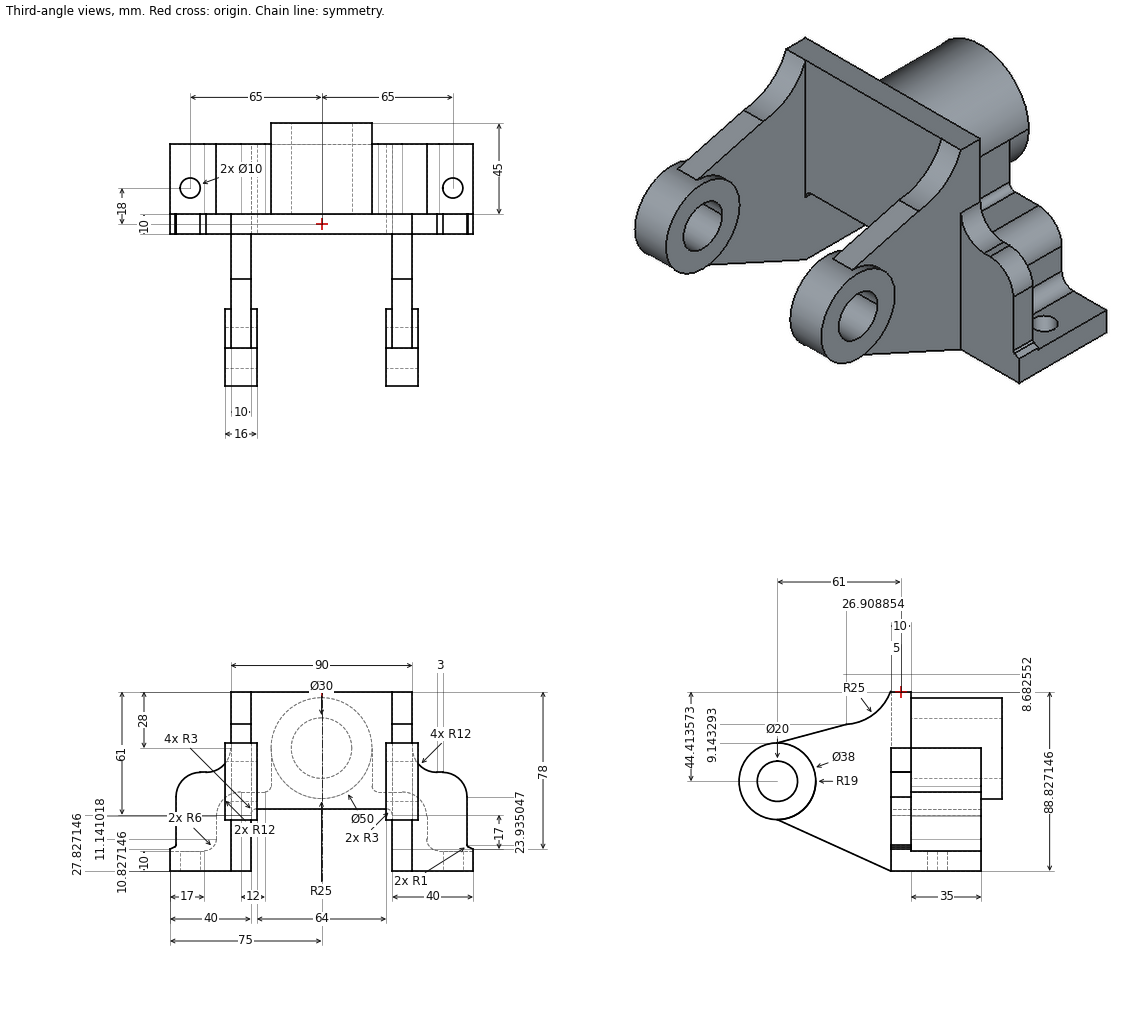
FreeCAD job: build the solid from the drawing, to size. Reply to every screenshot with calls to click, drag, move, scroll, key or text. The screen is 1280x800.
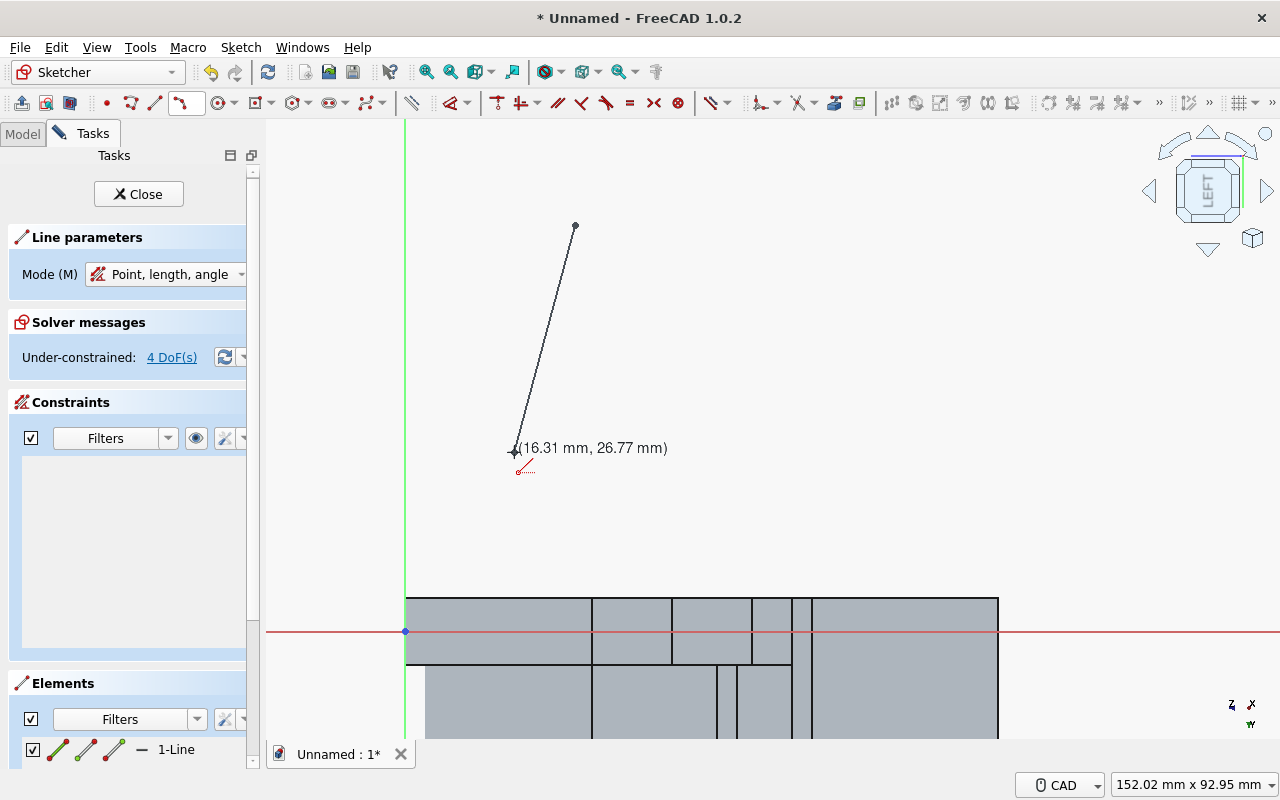
key(g)
key(m)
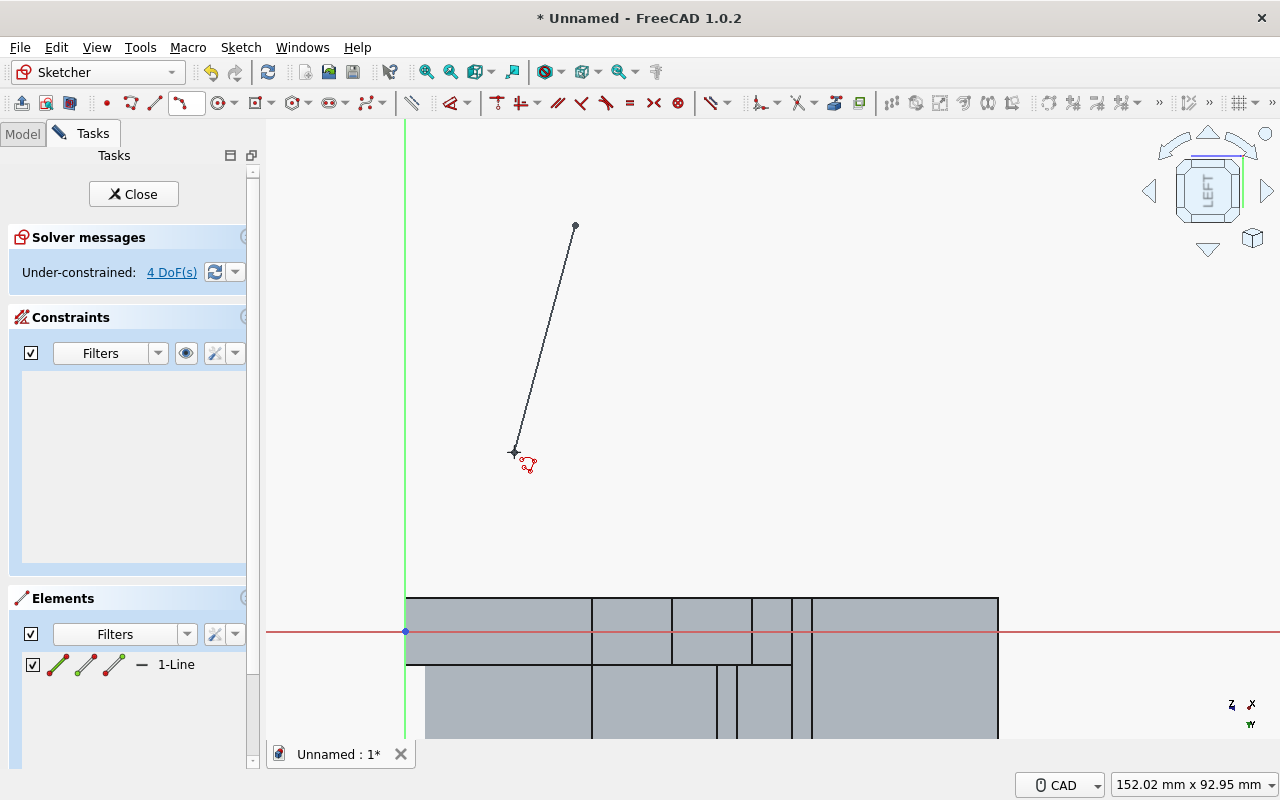
click(405, 598)
click(998, 598)
click(828, 225)
right_click(828, 225)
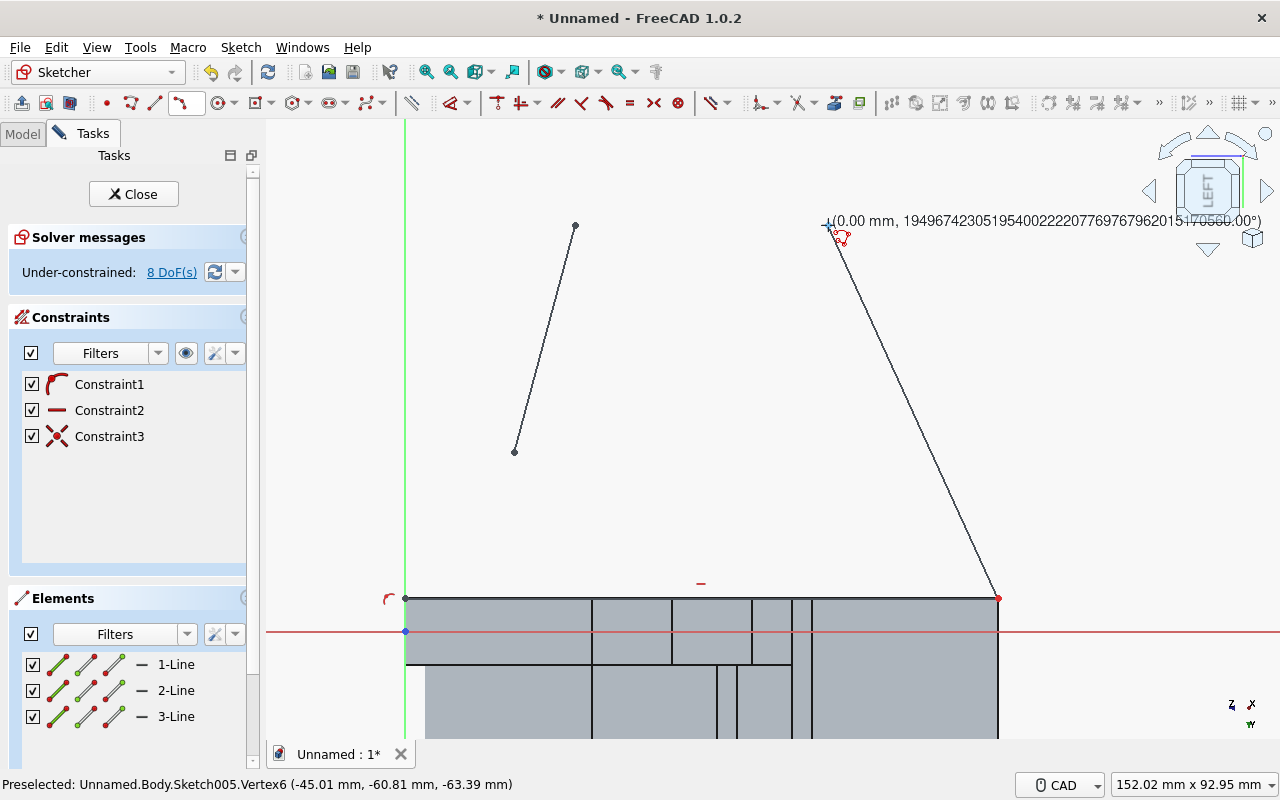
key(g)
key(3)
key(a)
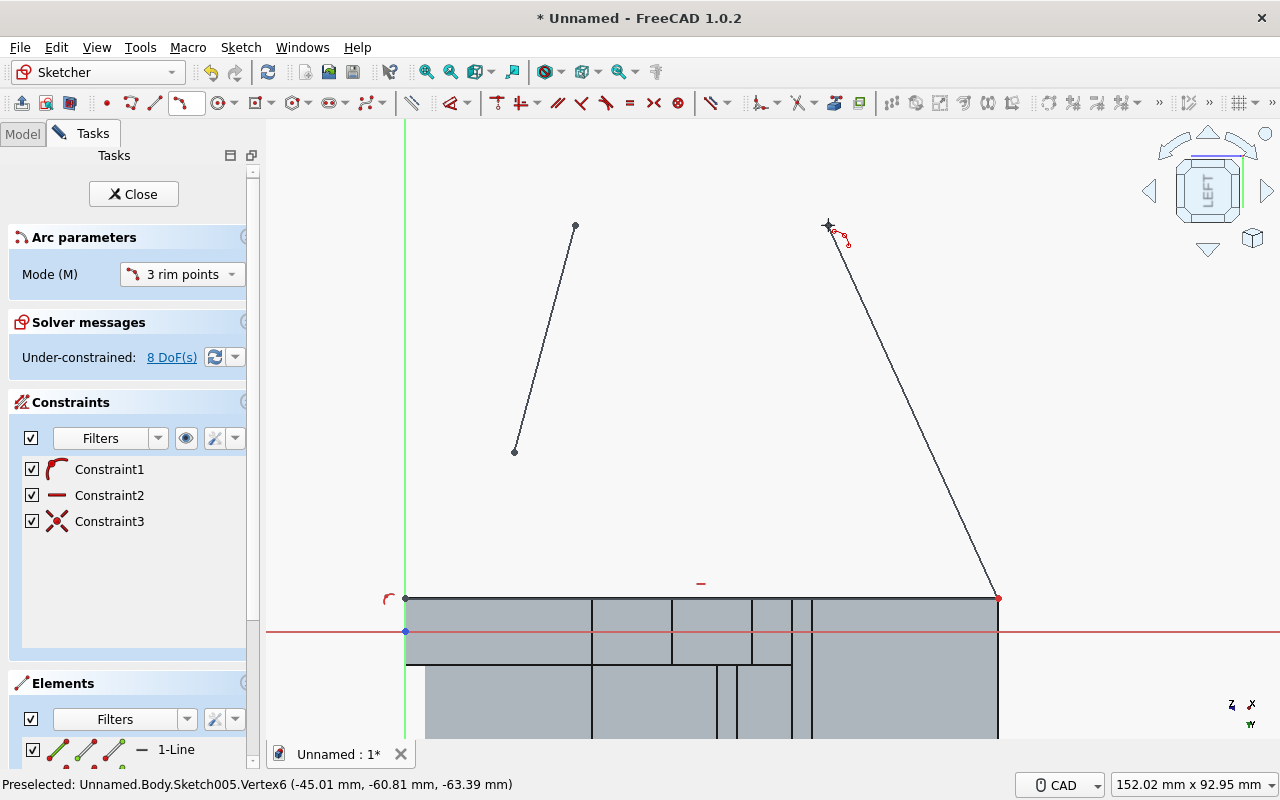
click(514, 453)
click(405, 599)
click(481, 541)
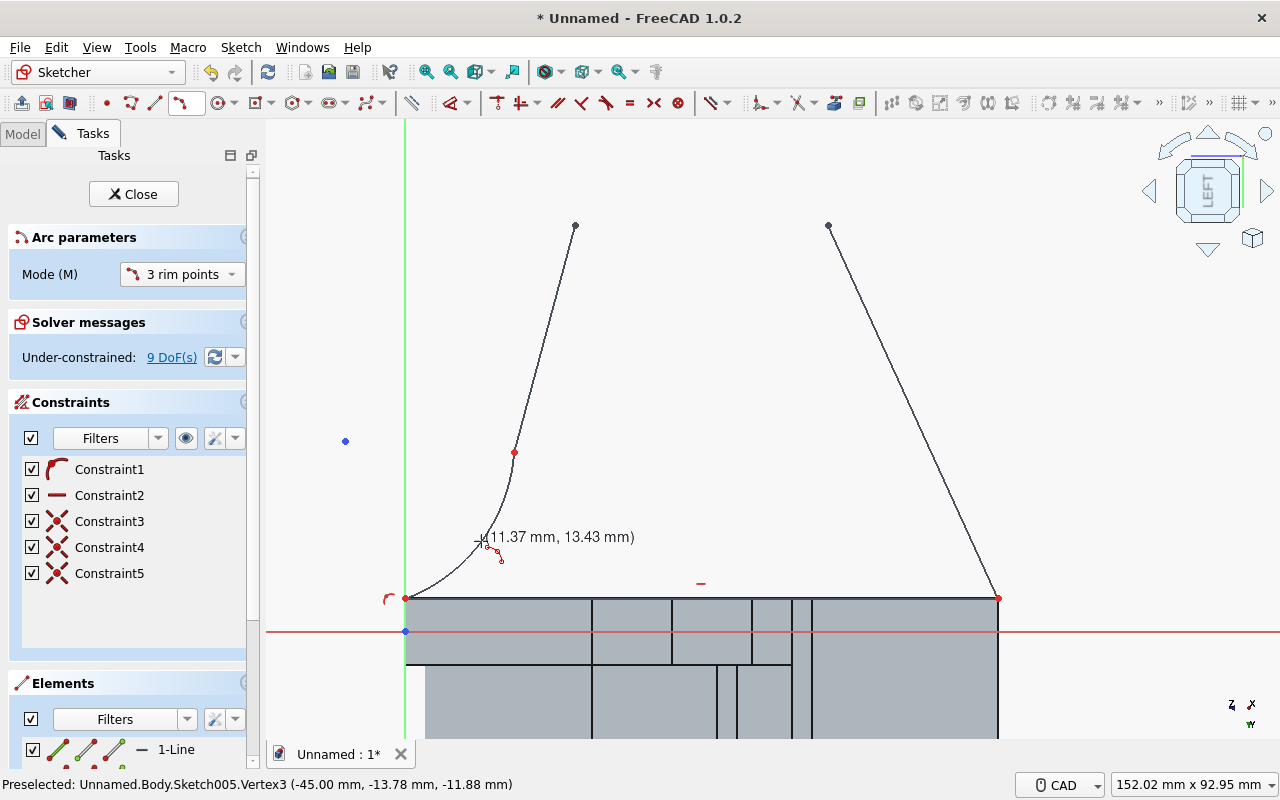
click(828, 226)
click(575, 226)
click(701, 351)
key(Escape)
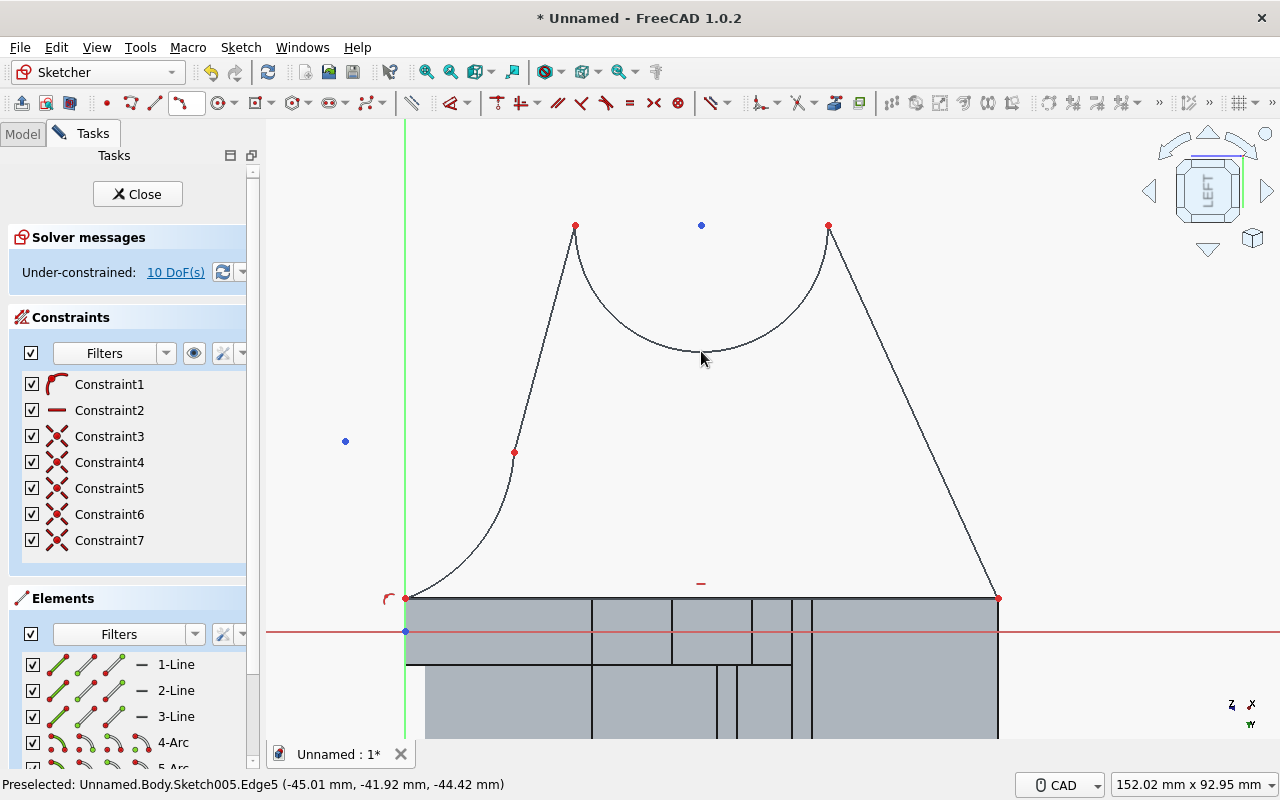
key(d)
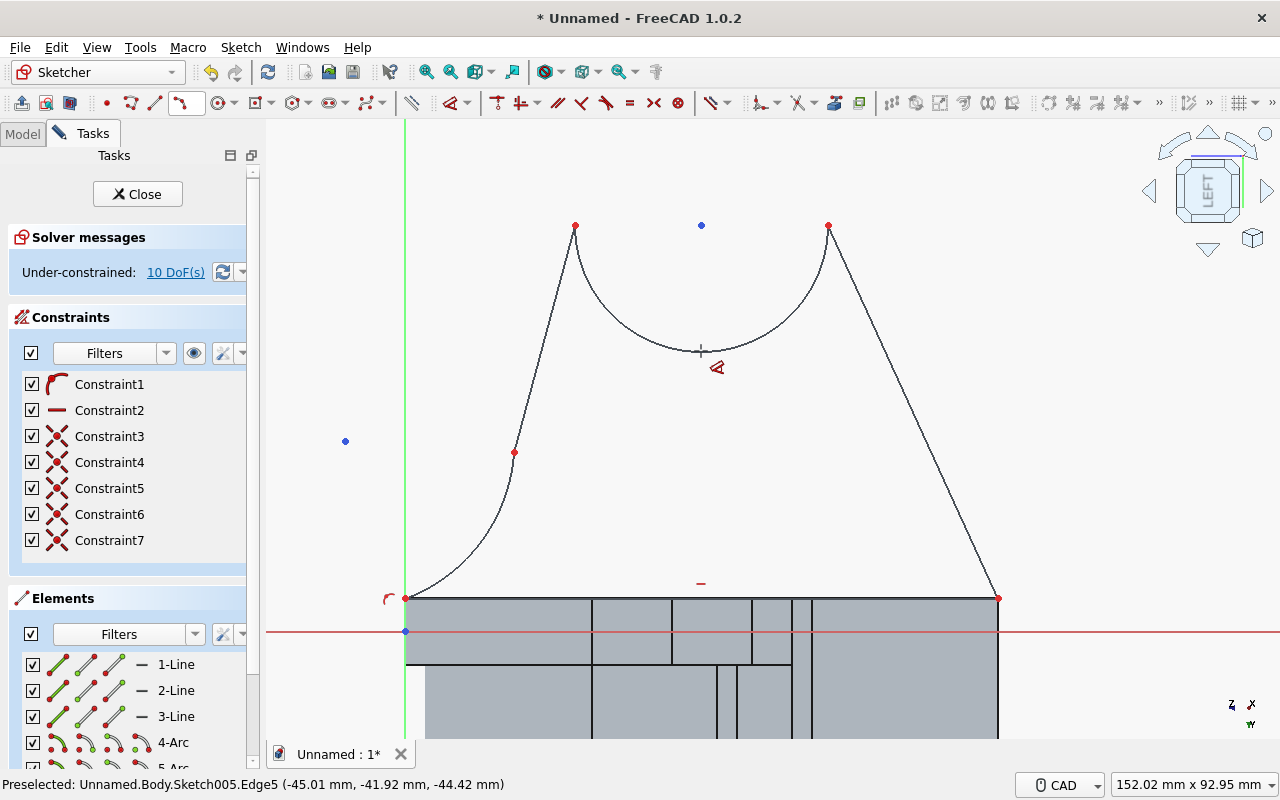
click(455, 570)
click(533, 513)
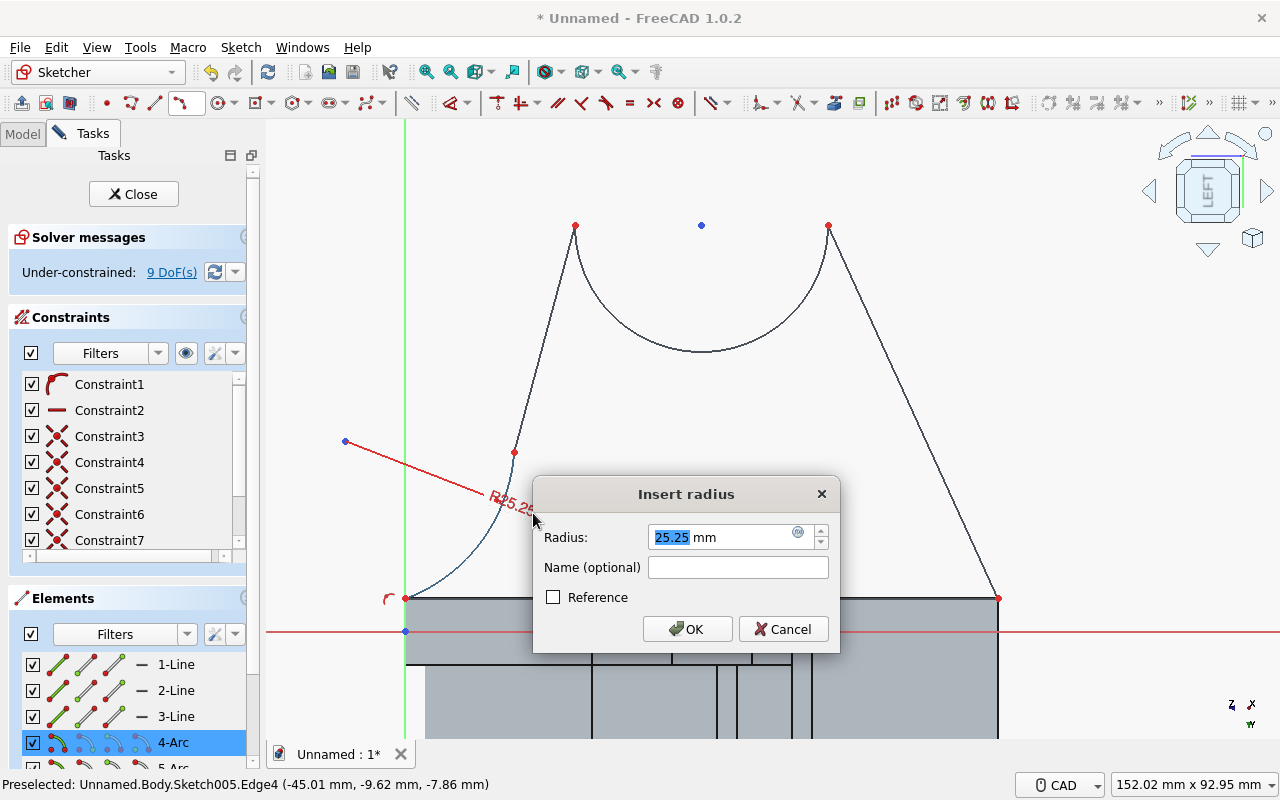
text(25)
key(Return)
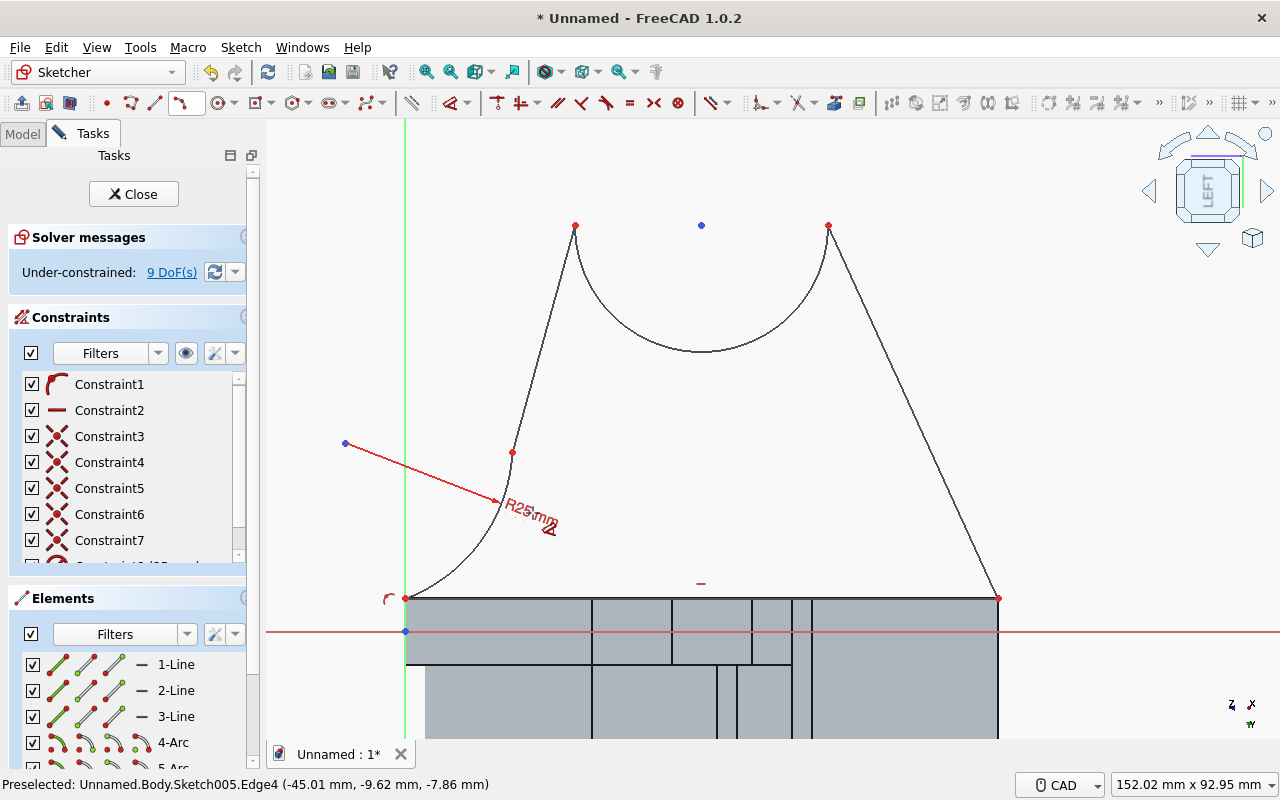
click(627, 328)
click(608, 354)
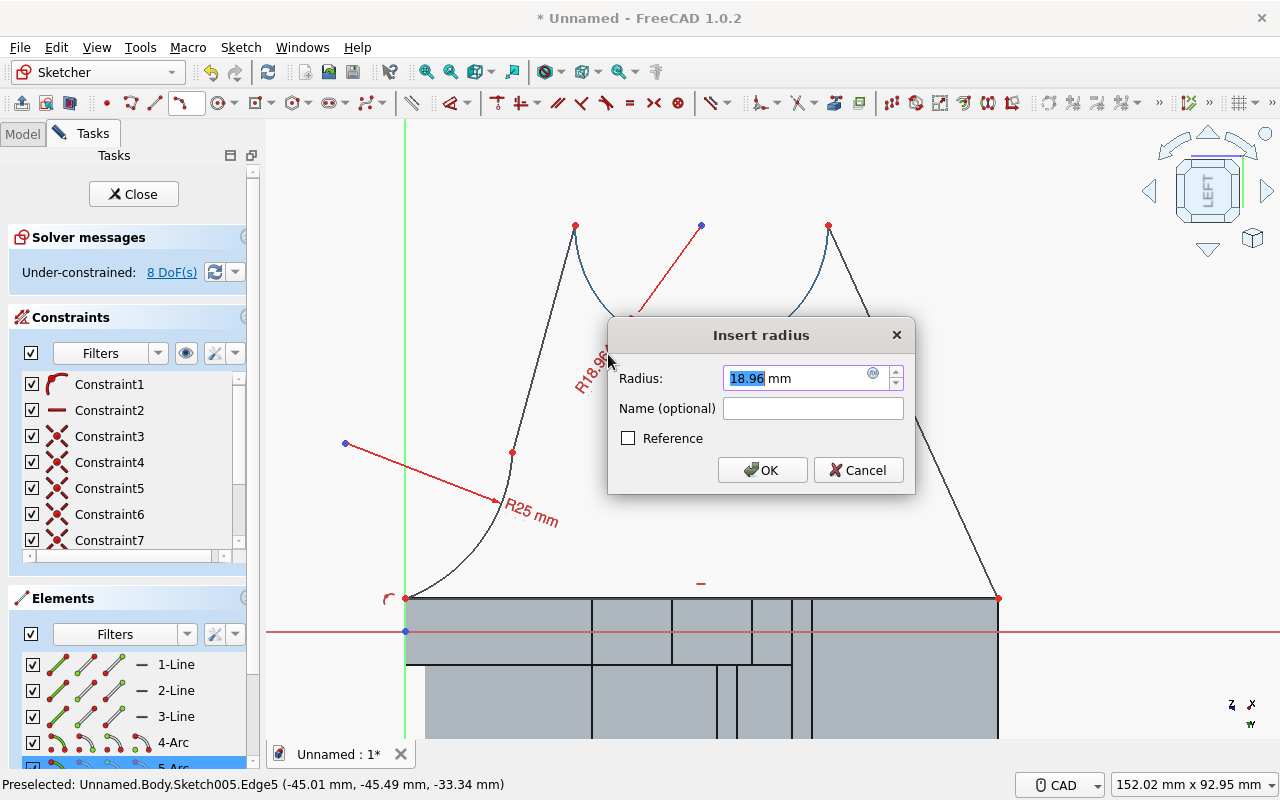
text(19)
key(Return)